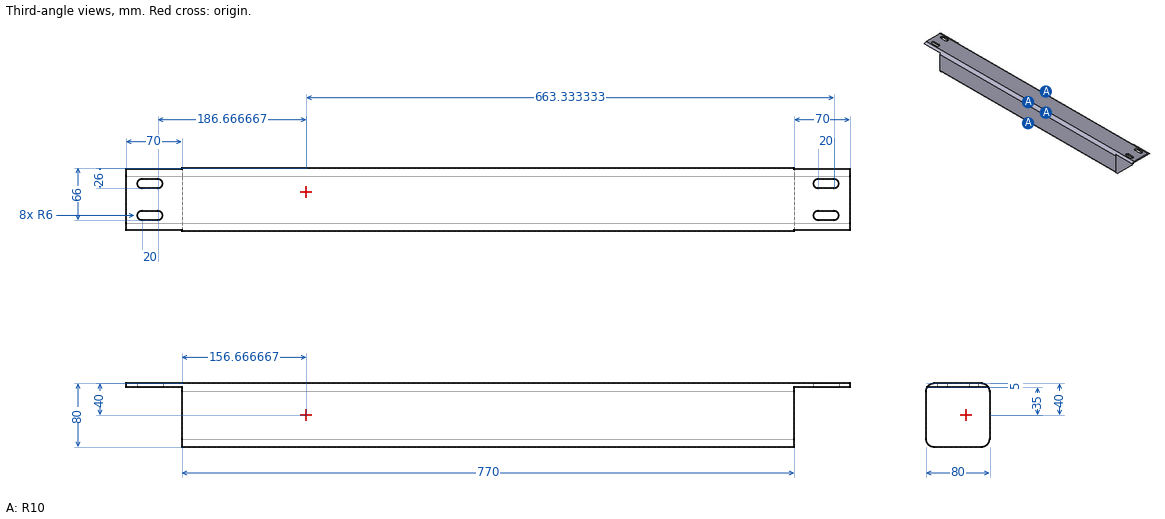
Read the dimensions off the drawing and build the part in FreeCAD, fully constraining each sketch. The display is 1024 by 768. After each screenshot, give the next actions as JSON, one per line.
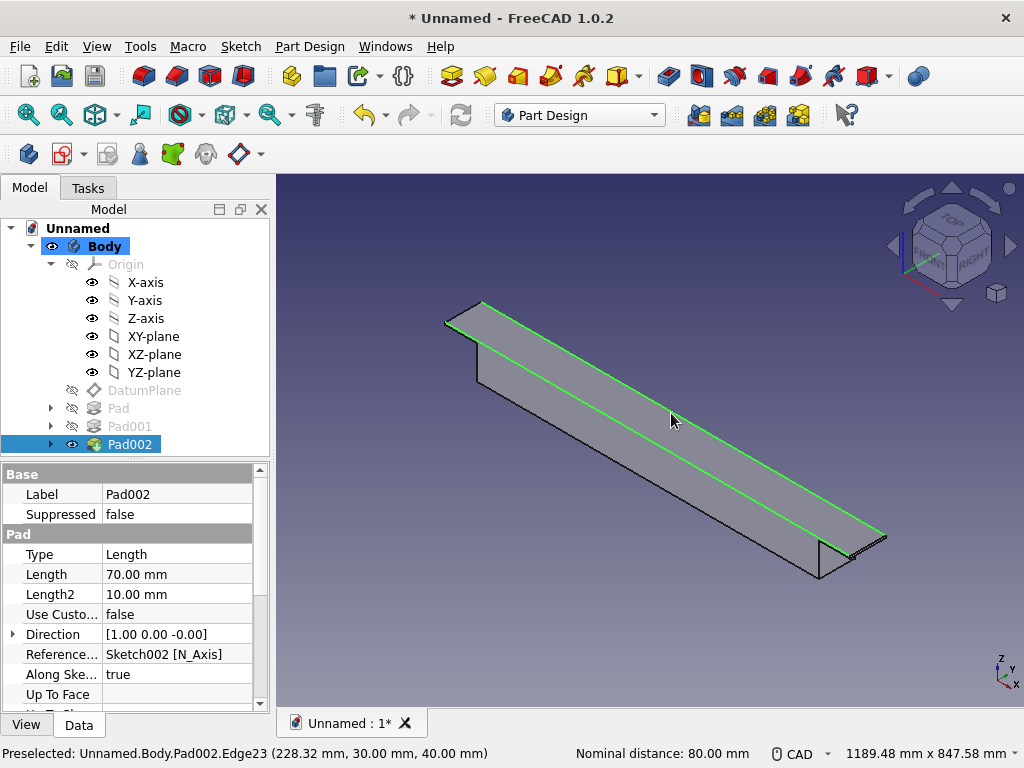
{"action": "key", "text": "1"}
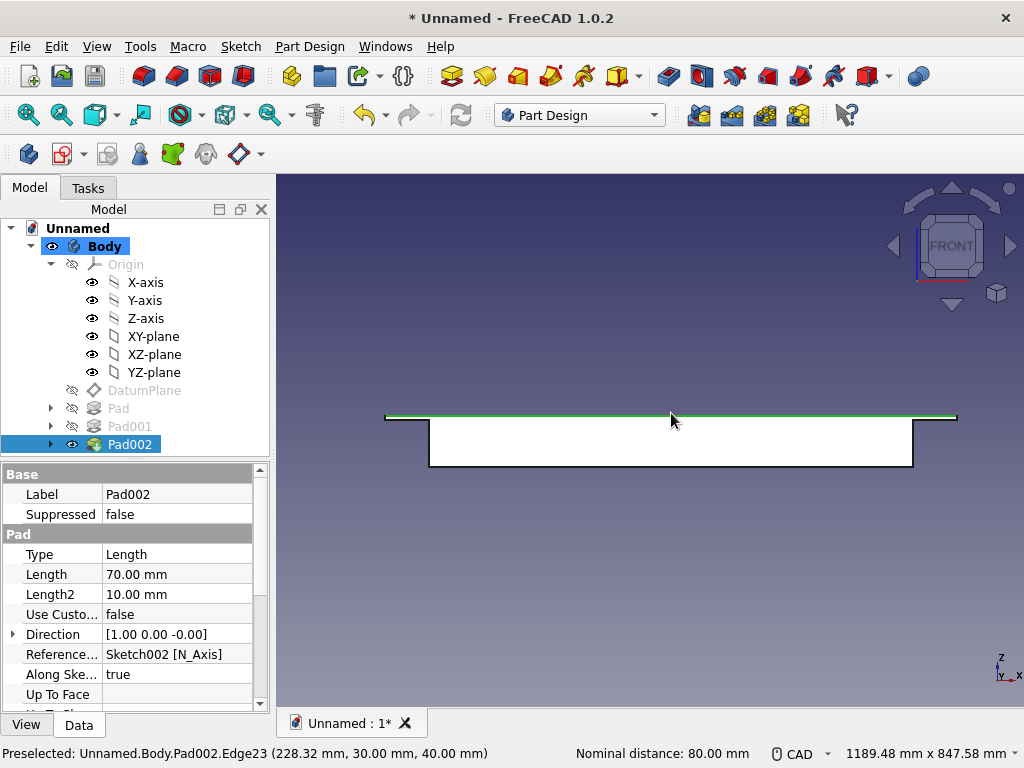
{"action": "key", "text": "3"}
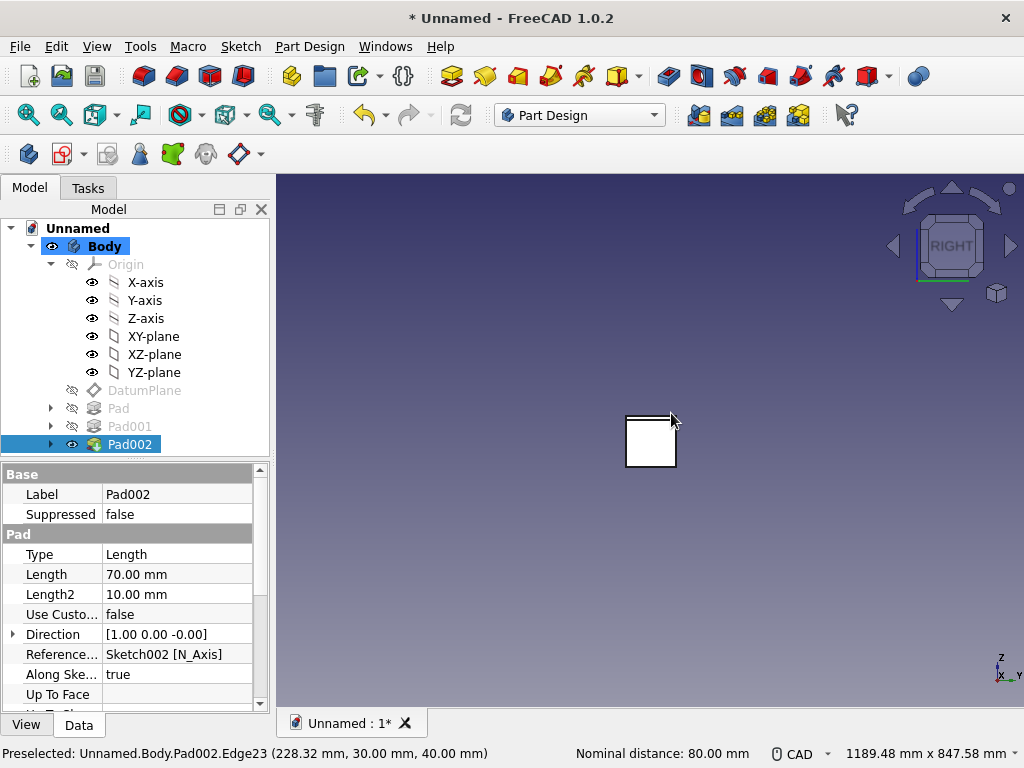
{"action": "left_click", "coordinate": [29, 116]}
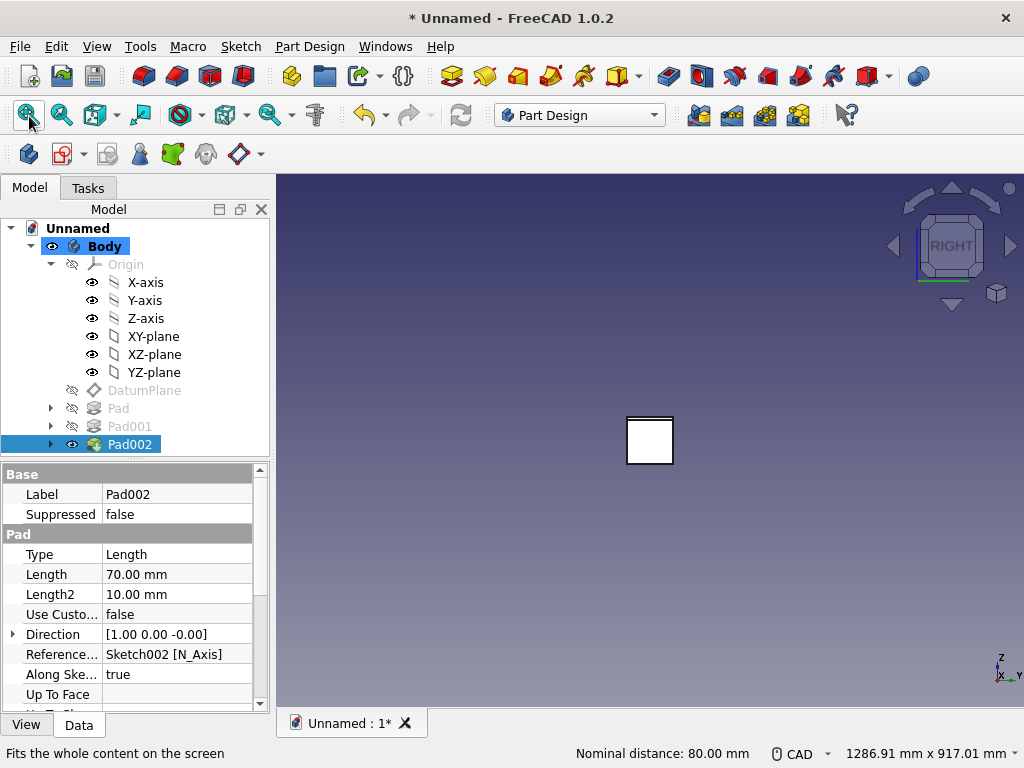
{"action": "key", "text": "5"}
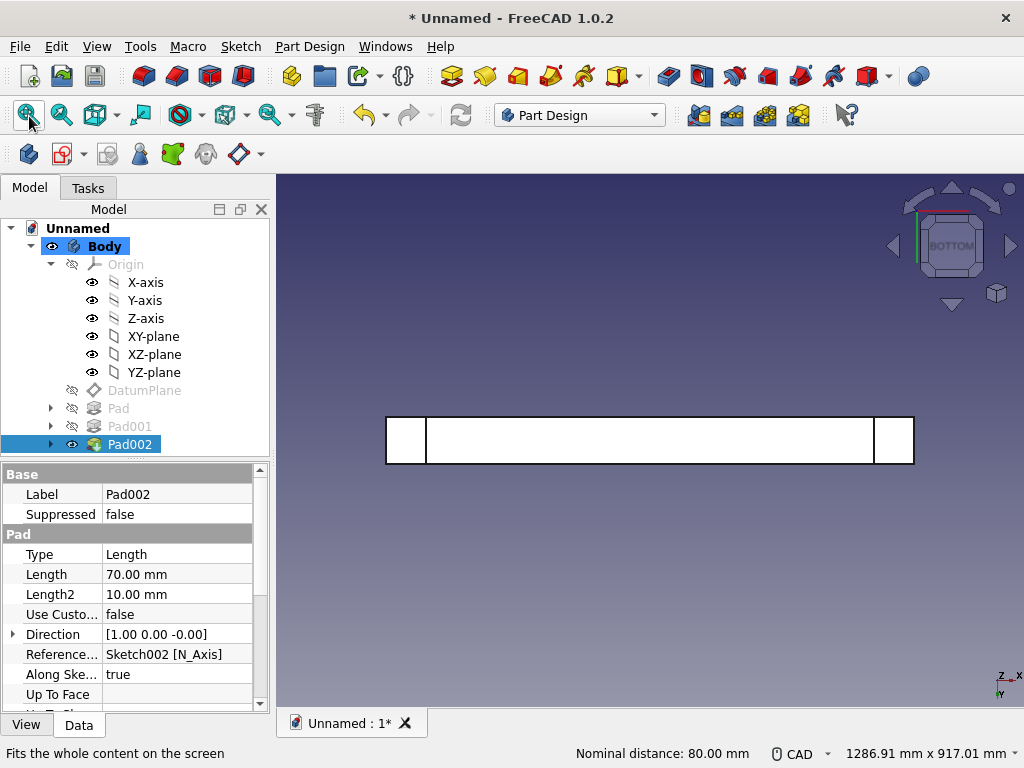
{"action": "left_click", "coordinate": [650, 416], "text": "ctrl"}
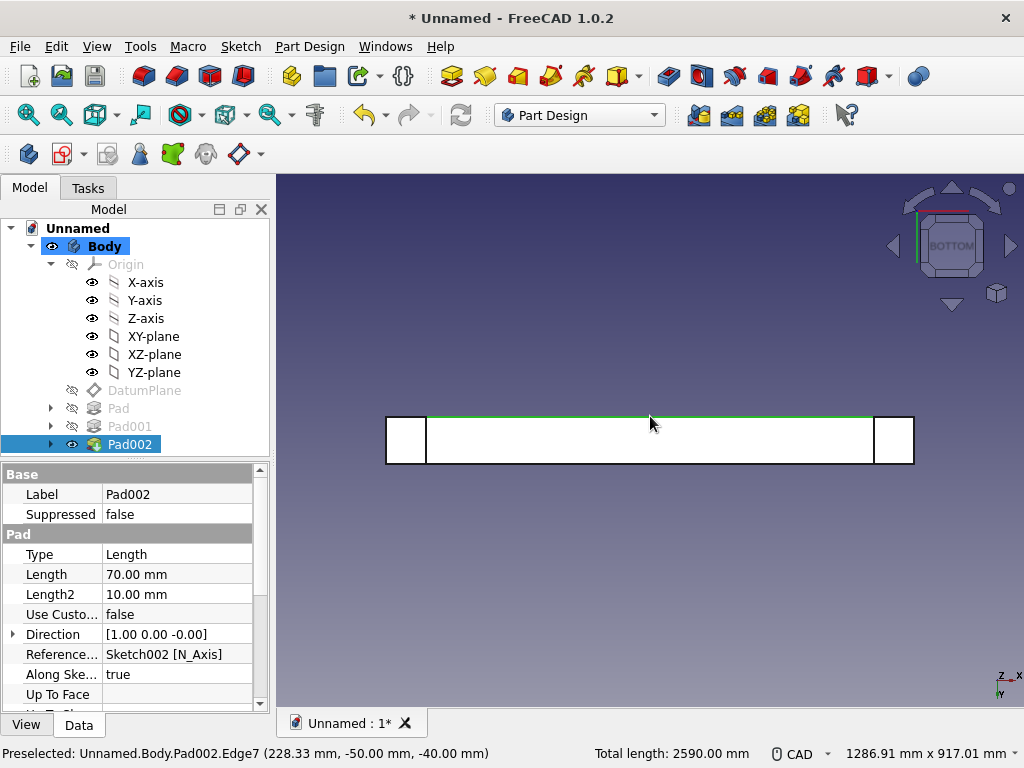
{"action": "key", "text": "4"}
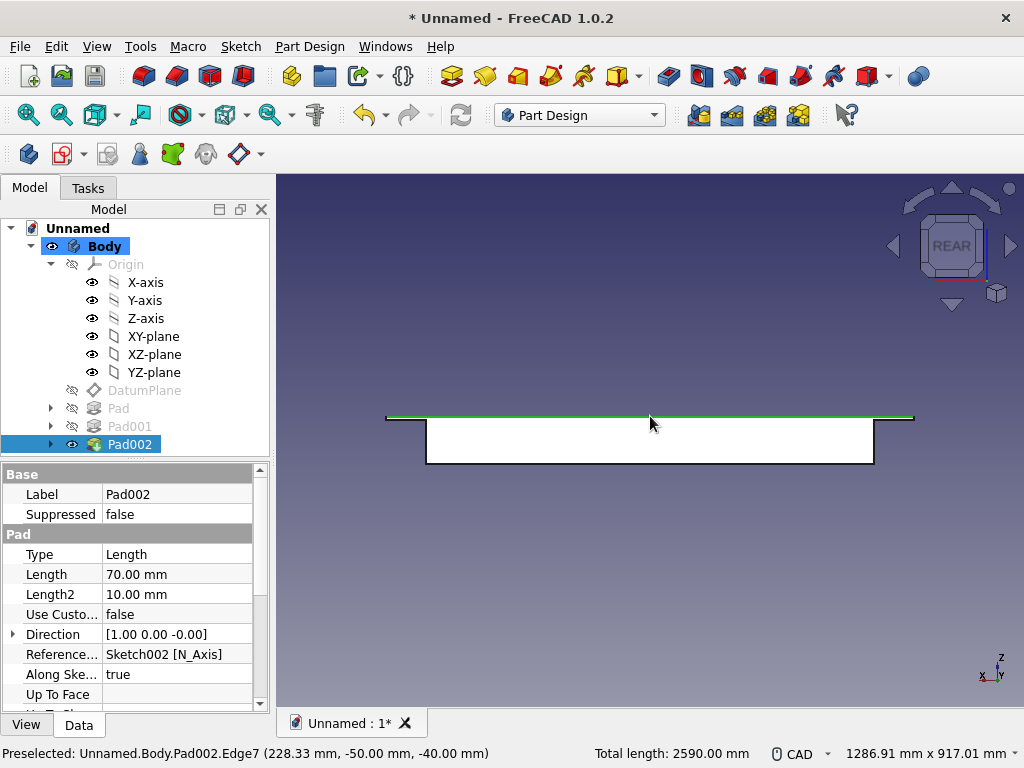
{"action": "left_click", "coordinate": [650, 463], "text": "ctrl"}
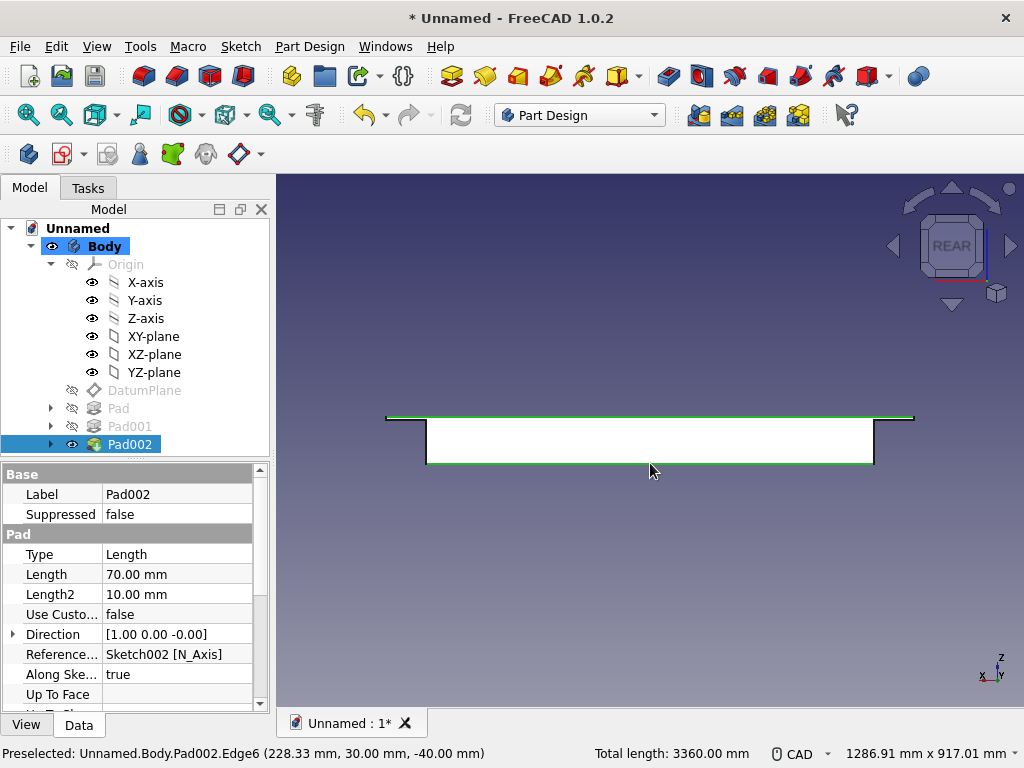
{"action": "left_click", "coordinate": [144, 76]}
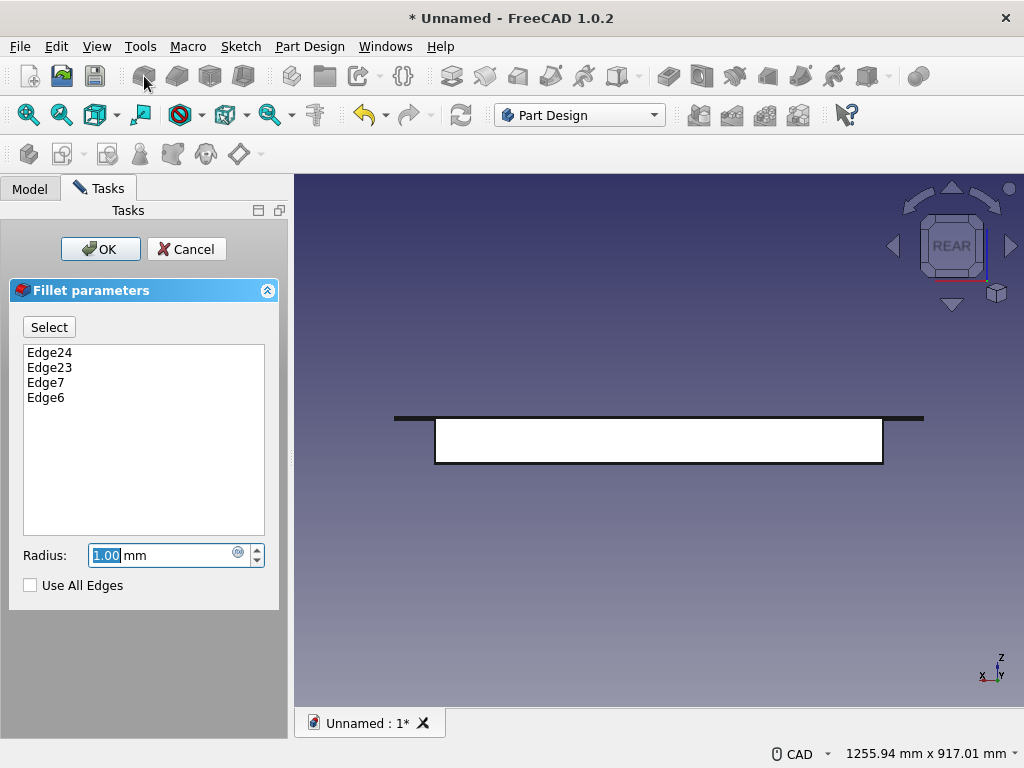
{"action": "type", "text": "10"}
{"action": "key", "text": "Tab"}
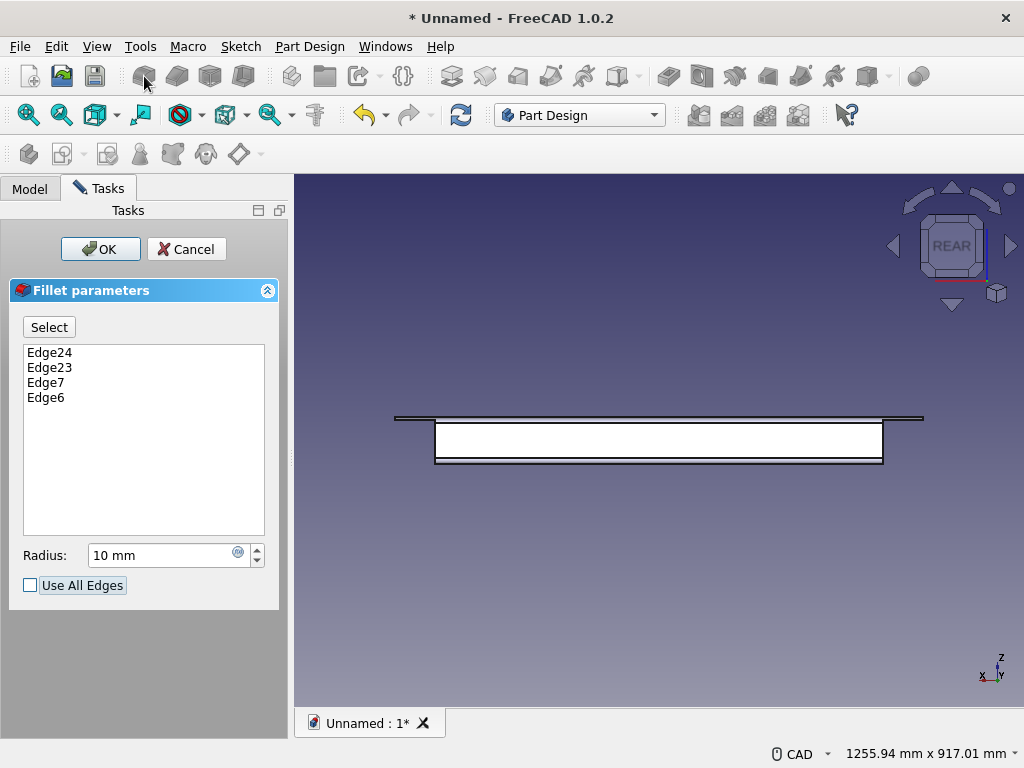
{"action": "left_click", "coordinate": [101, 249]}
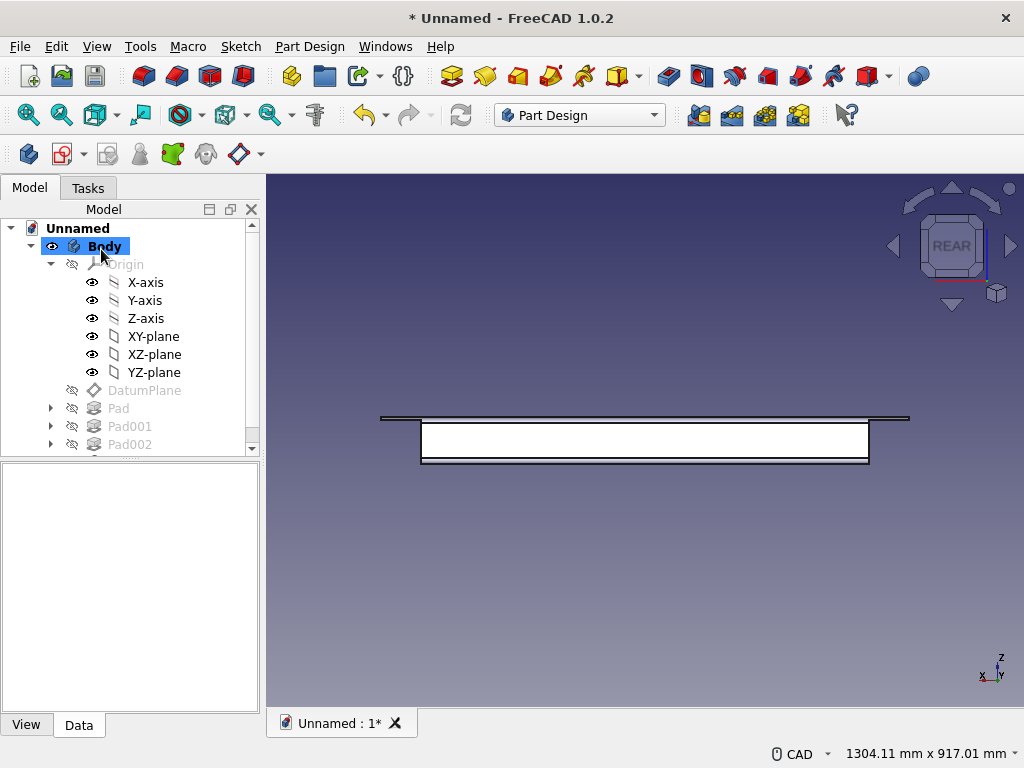
{"action": "key", "text": "0"}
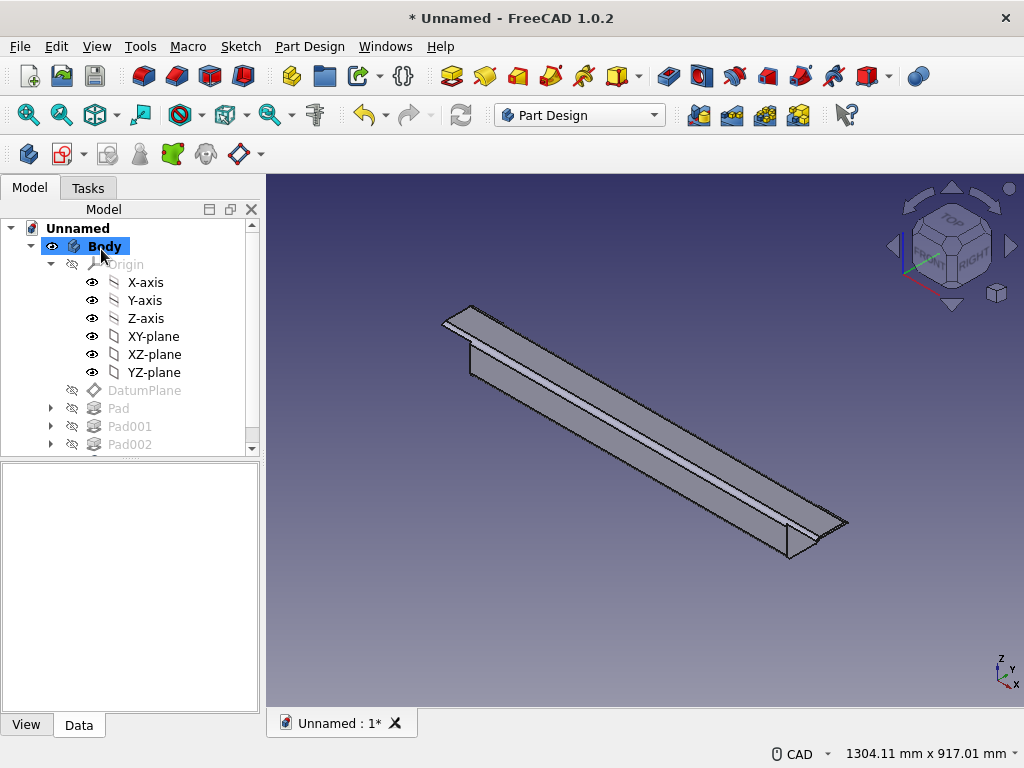
{"action": "left_click", "coordinate": [752, 482]}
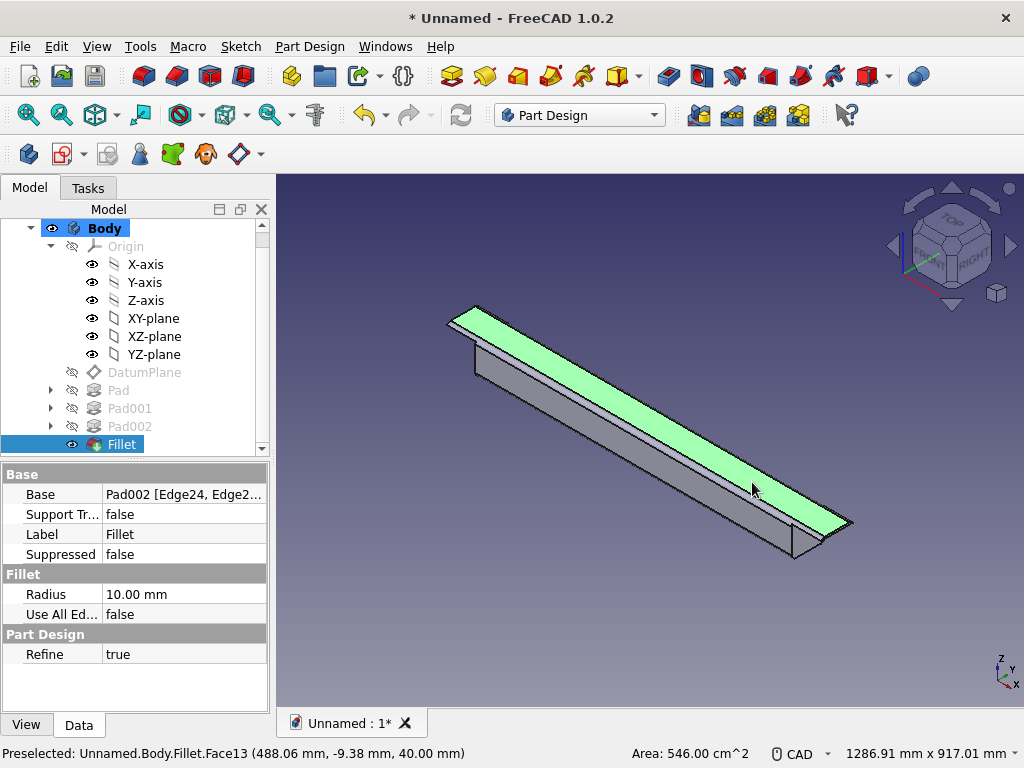
{"action": "left_click", "coordinate": [62, 154]}